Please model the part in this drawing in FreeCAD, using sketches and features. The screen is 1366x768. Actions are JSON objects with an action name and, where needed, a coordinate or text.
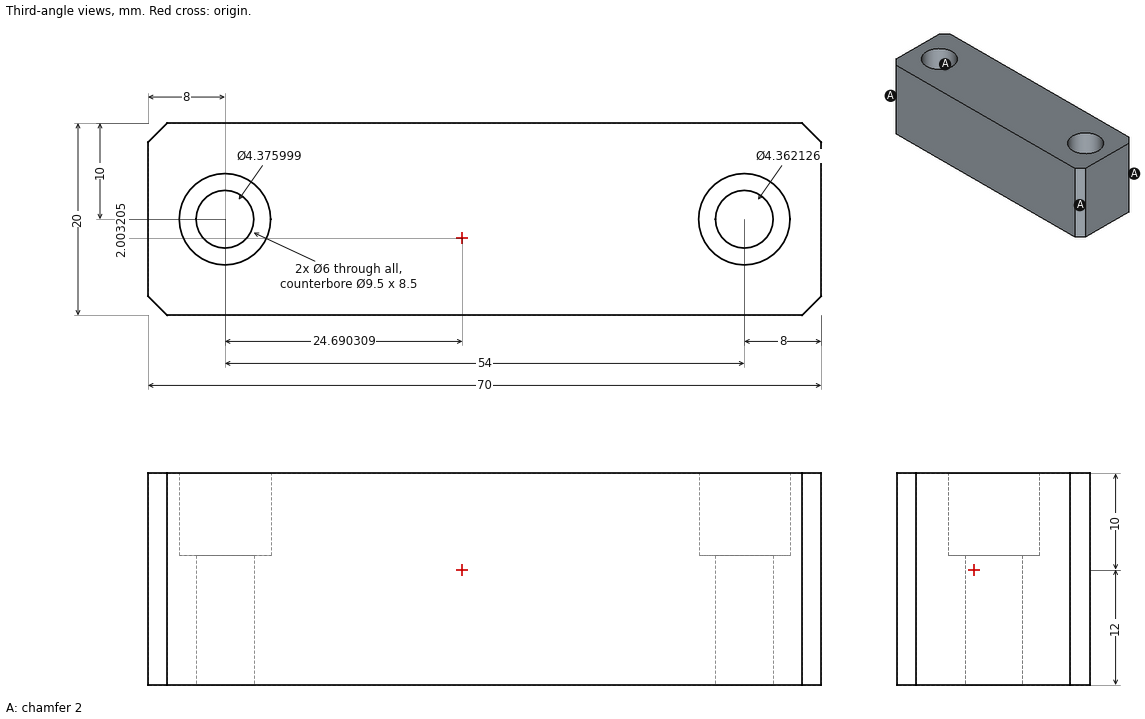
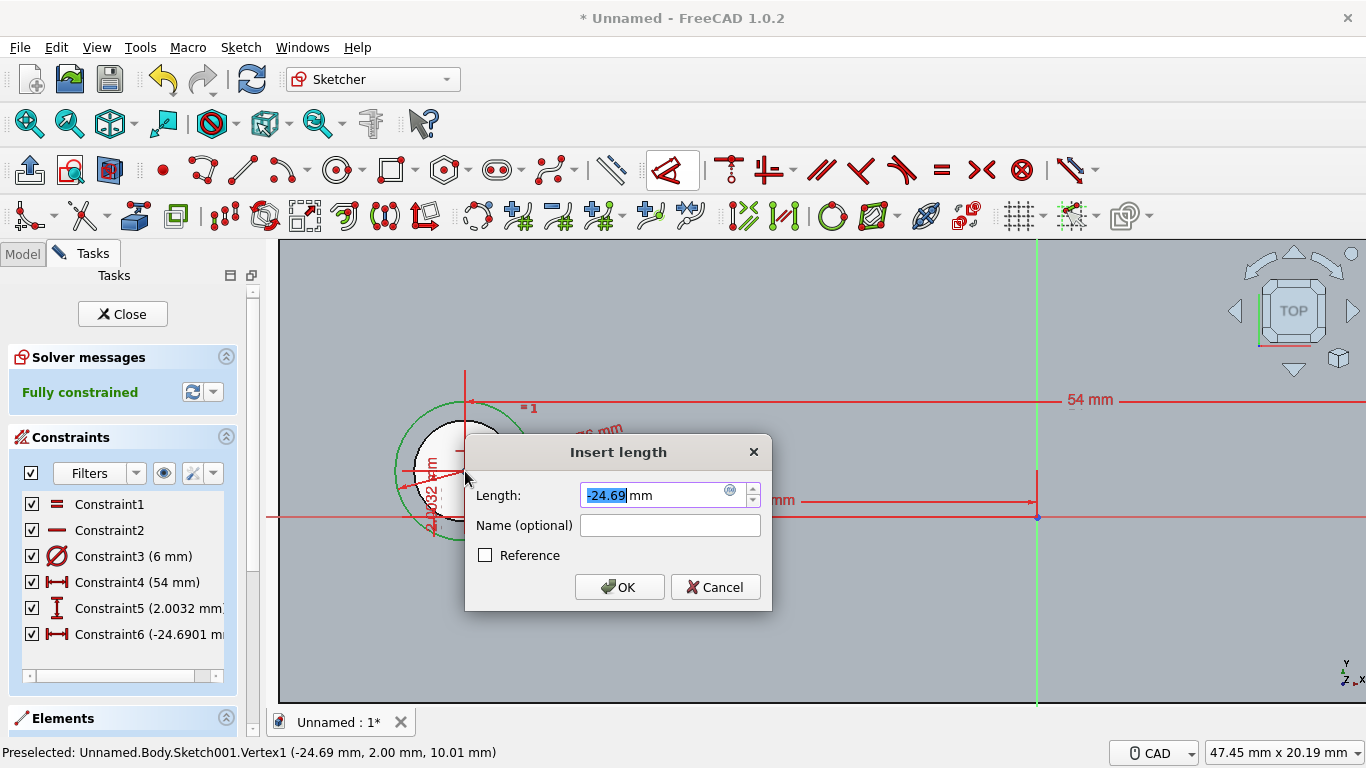
{"action": "type", "text": "-24.690309"}
{"action": "key", "text": "Return"}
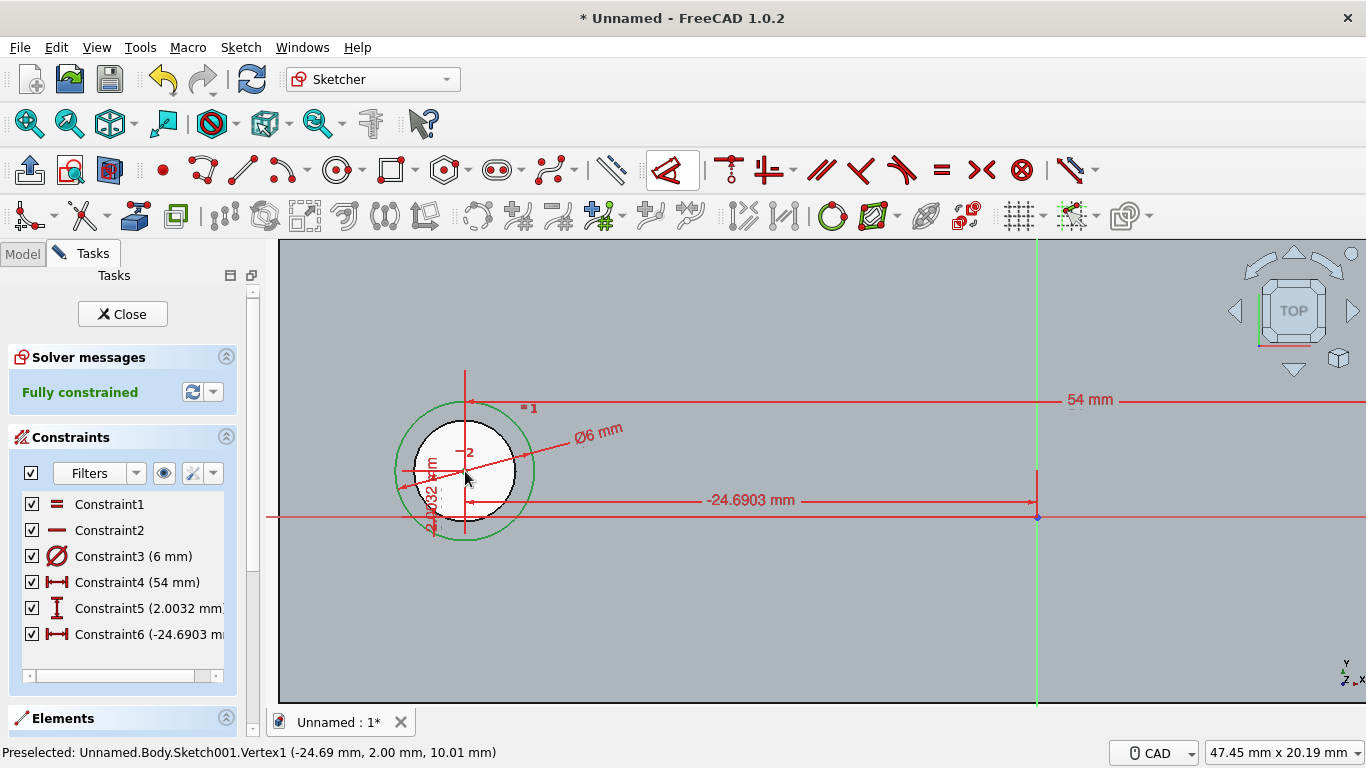
{"action": "left_click", "coordinate": [123, 314]}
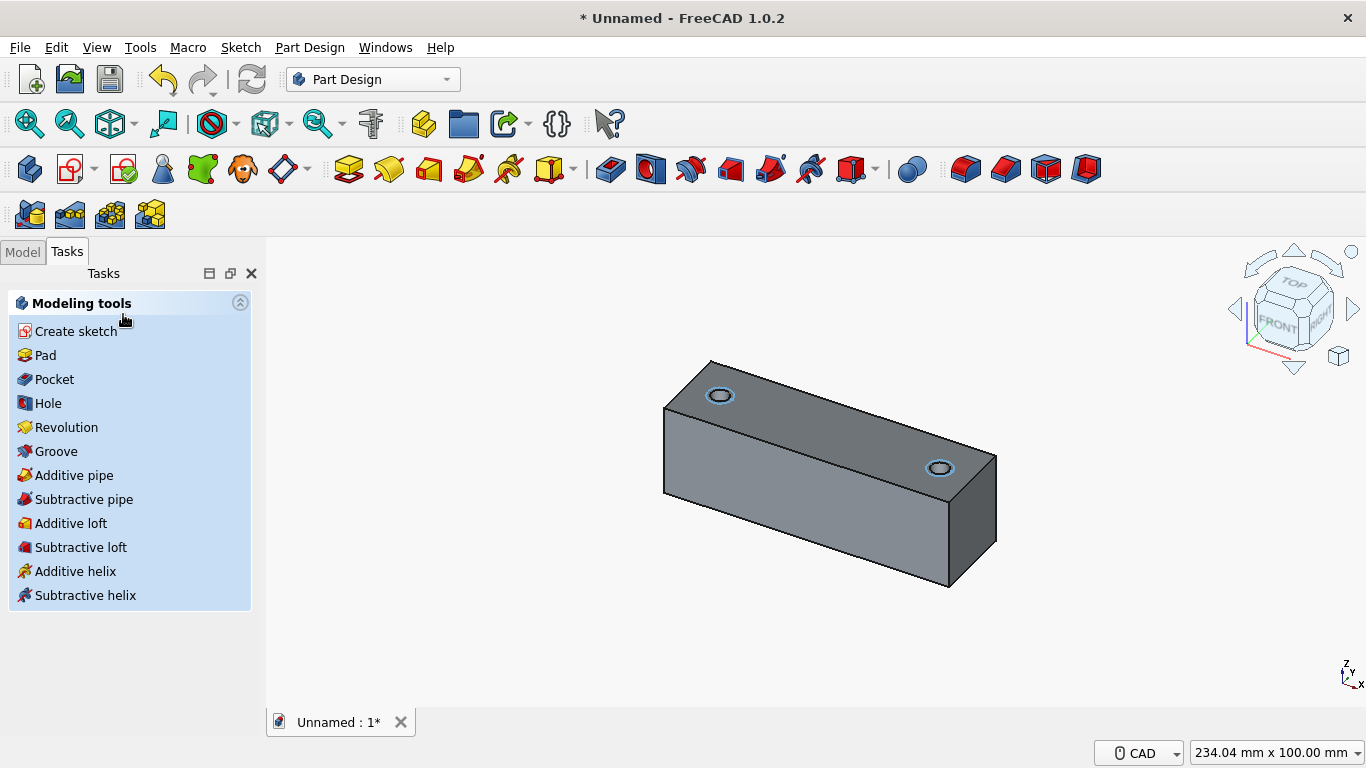
{"action": "left_click", "coordinate": [652, 170]}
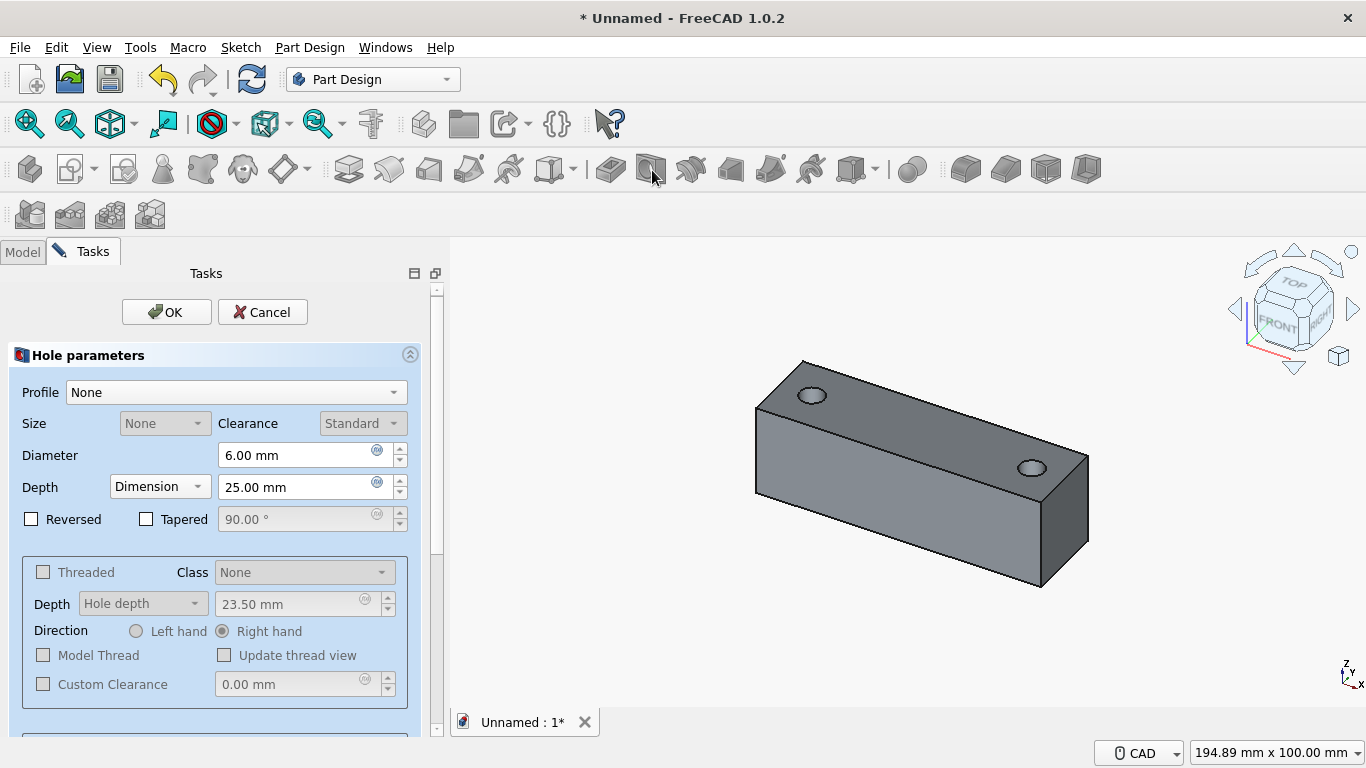
{"action": "triple_click", "coordinate": [305, 455]}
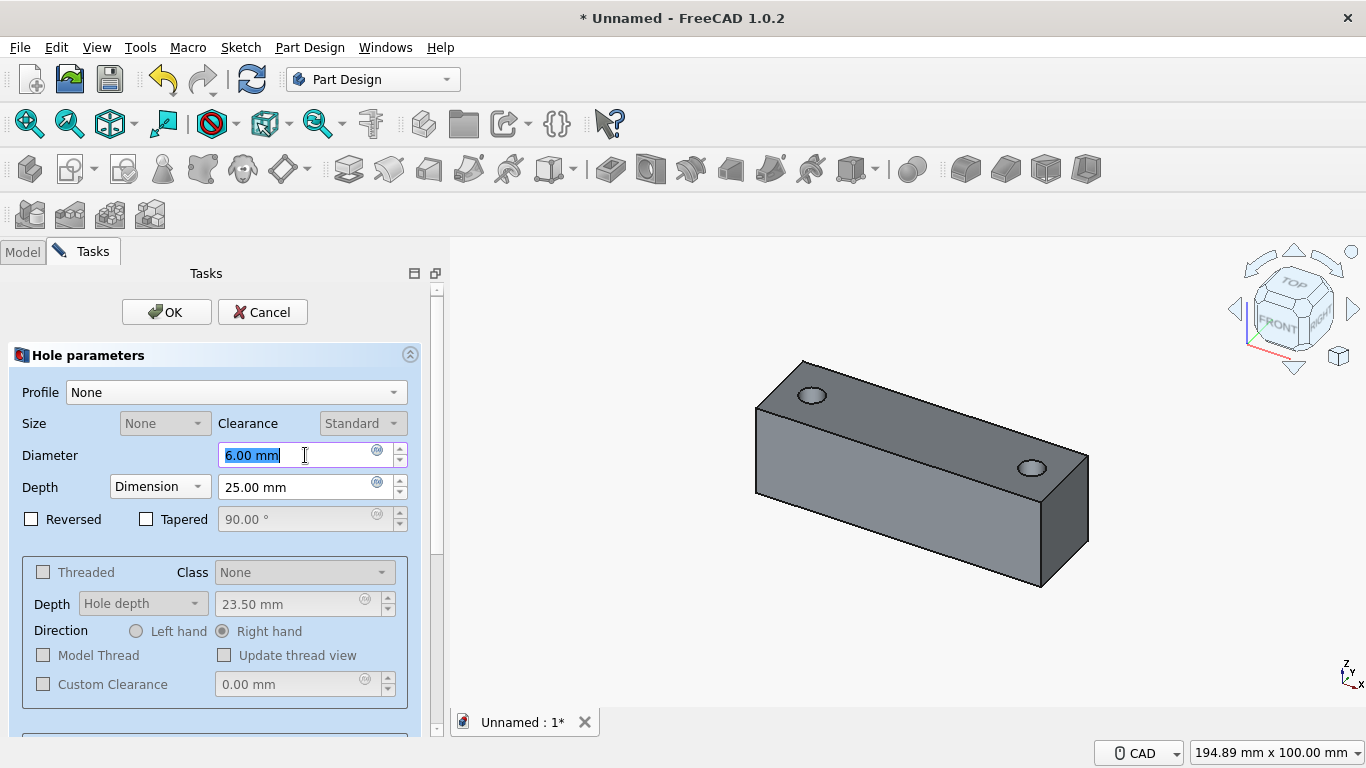
{"action": "type", "text": "6"}
{"action": "key", "text": "Tab"}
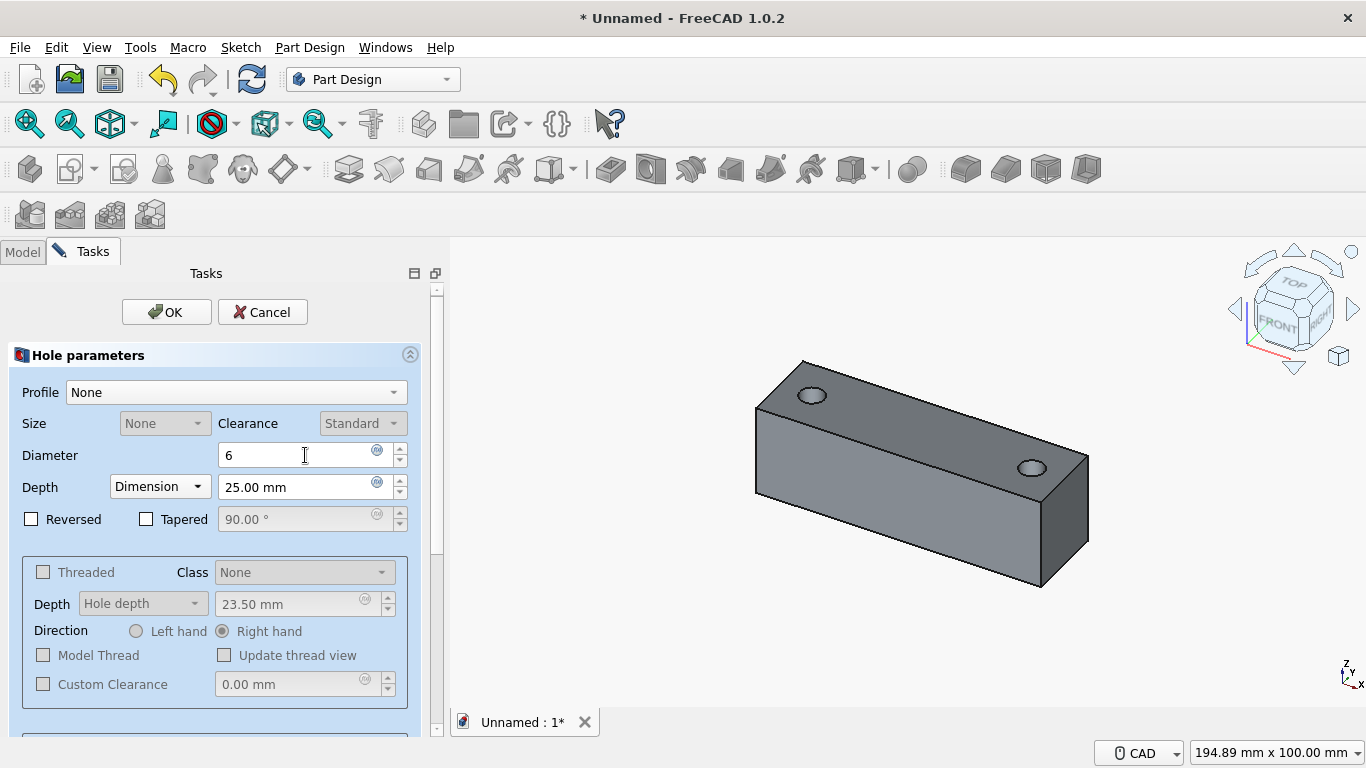
{"action": "left_click", "coordinate": [161, 486]}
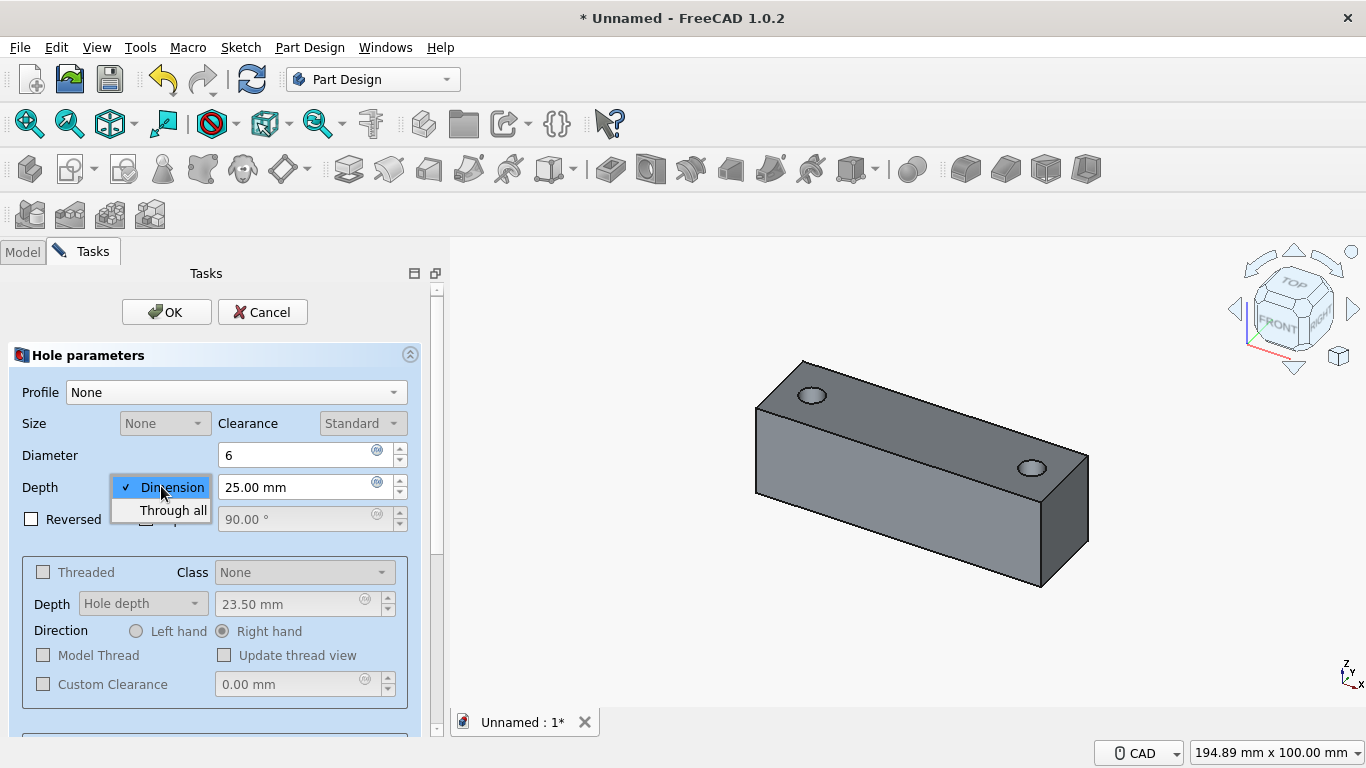
{"action": "left_click", "coordinate": [160, 510]}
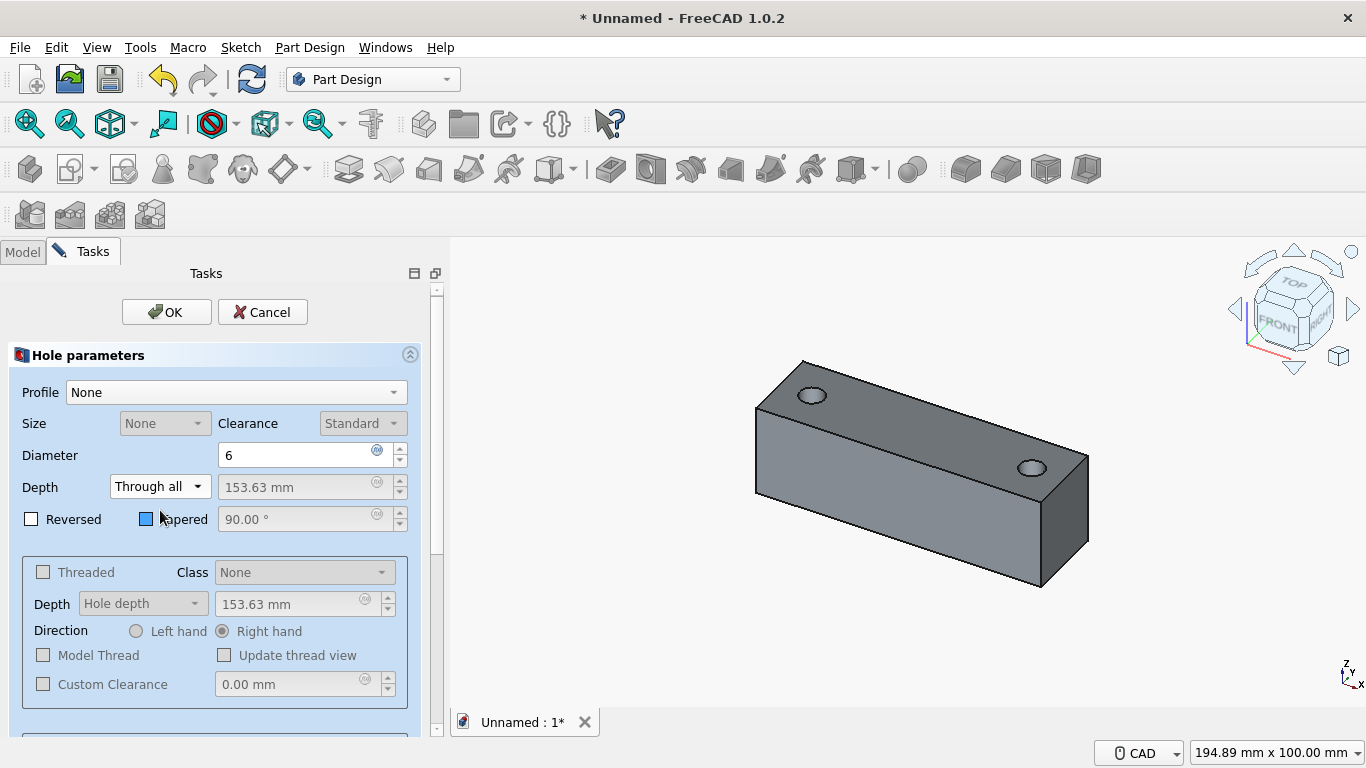
{"action": "scroll", "coordinate": [437, 510], "scroll_direction": "down", "scroll_amount": 2}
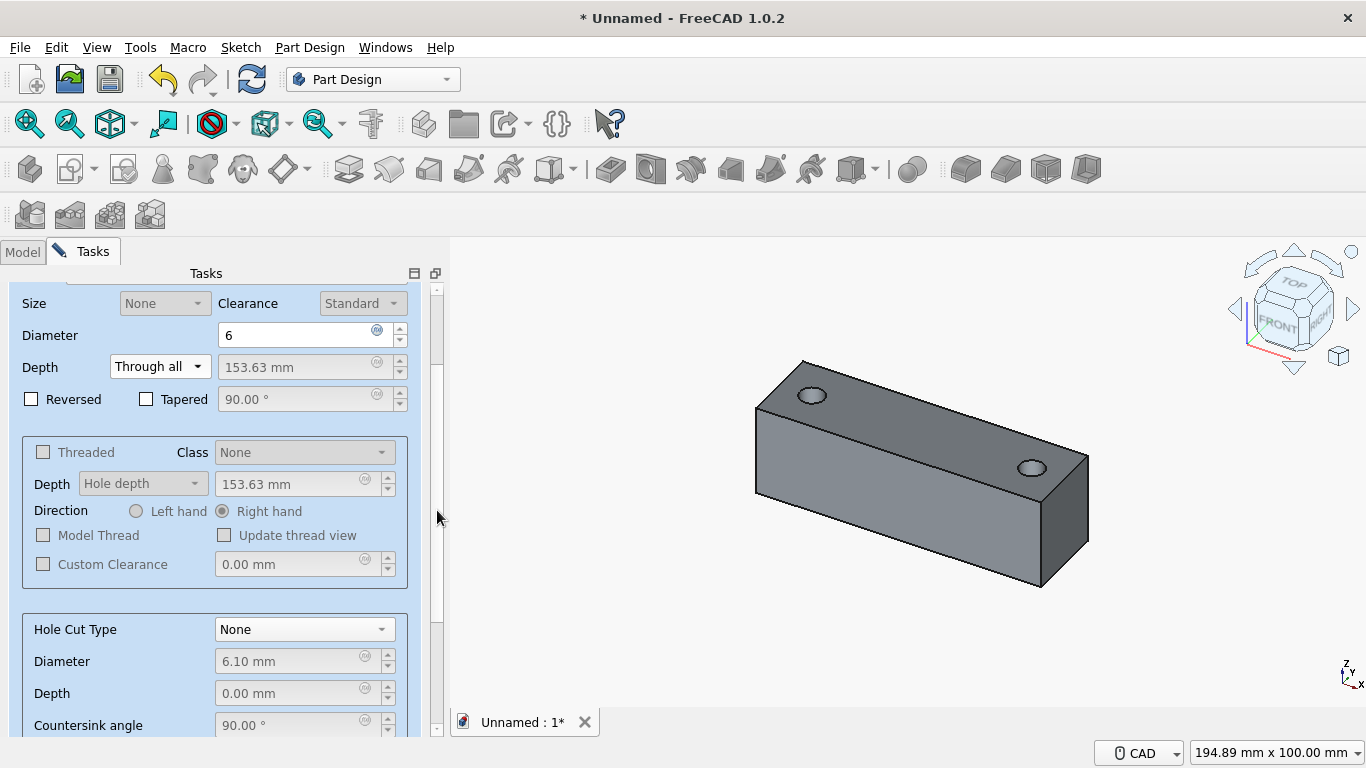
{"action": "left_click", "coordinate": [306, 630]}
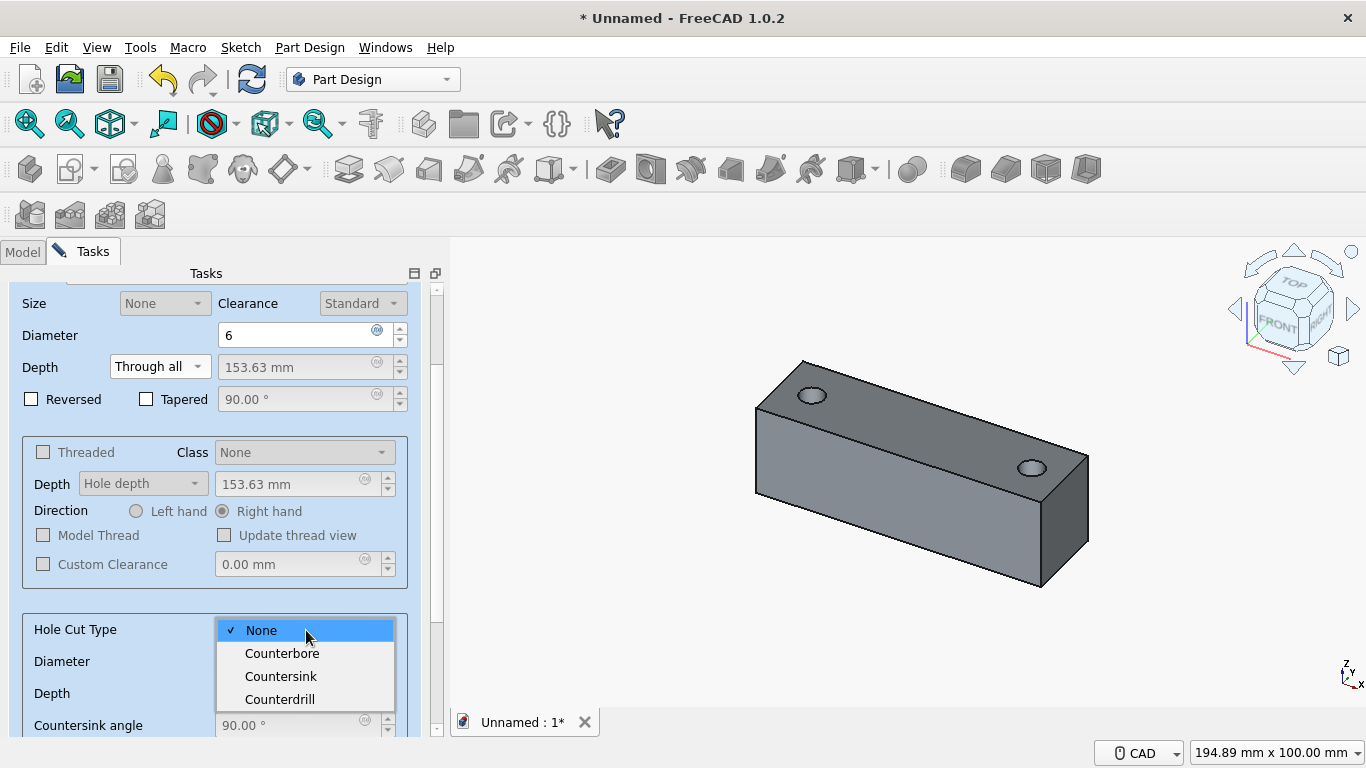
{"action": "left_click", "coordinate": [304, 654]}